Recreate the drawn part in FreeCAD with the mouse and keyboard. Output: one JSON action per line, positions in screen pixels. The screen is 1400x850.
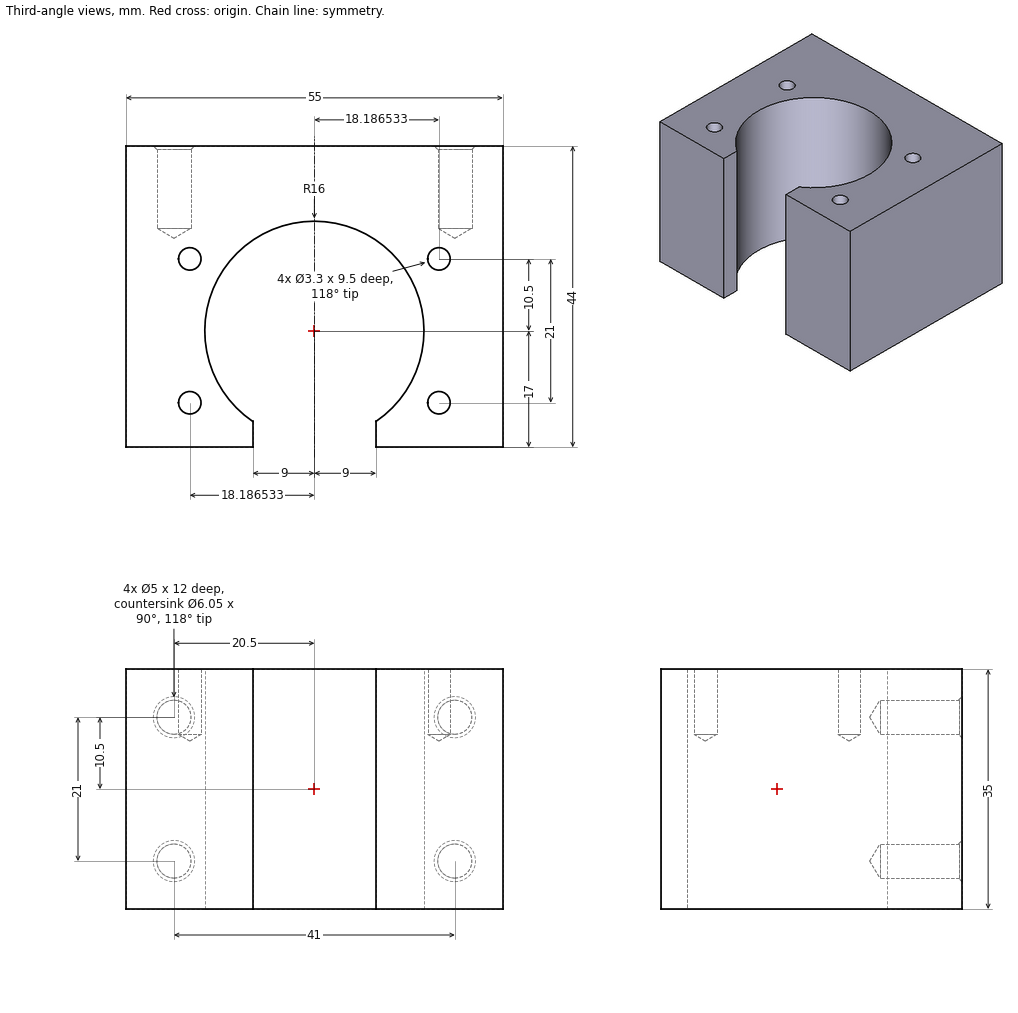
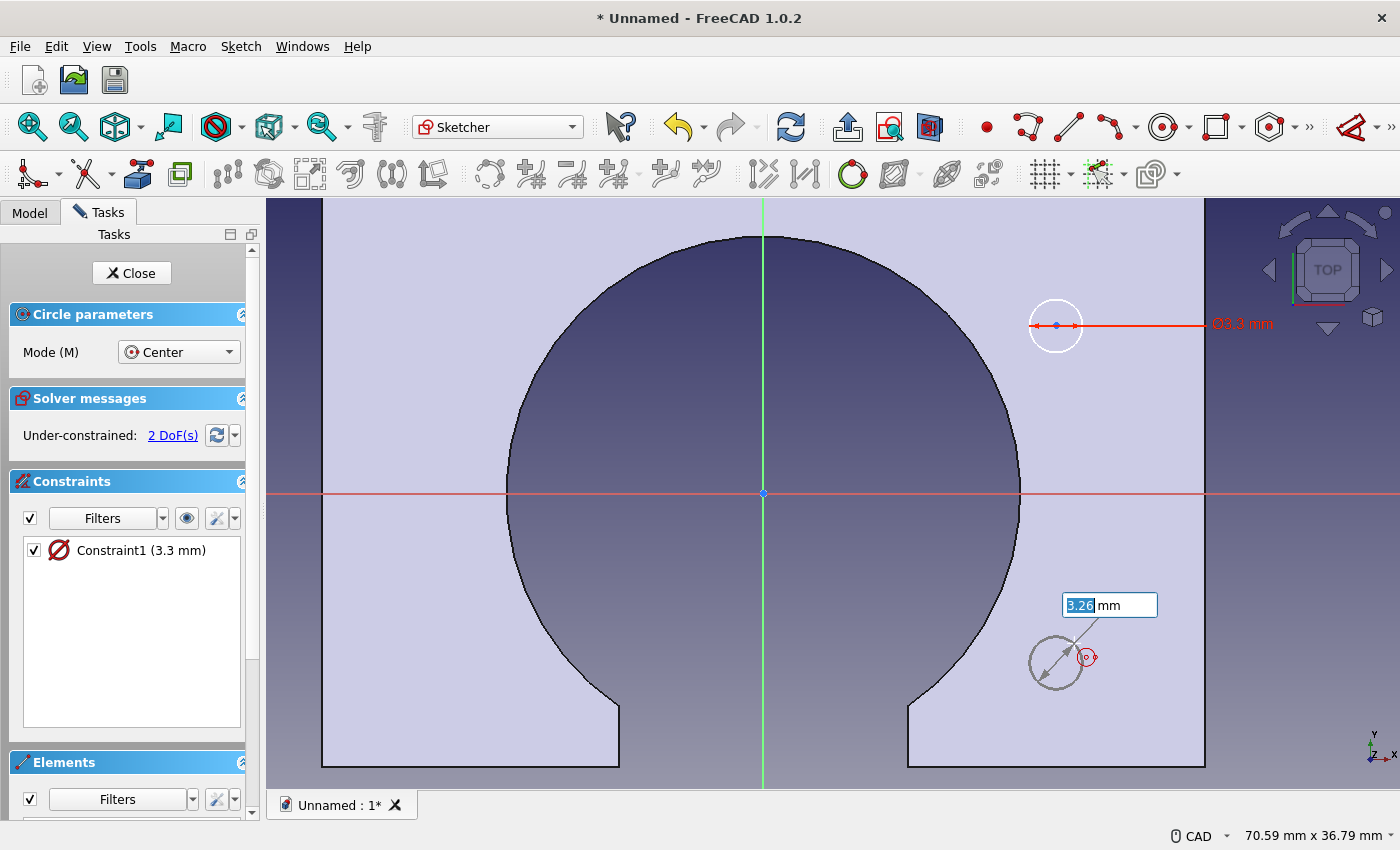
{"action": "type", "text": "3.3"}
{"action": "key", "text": "Return"}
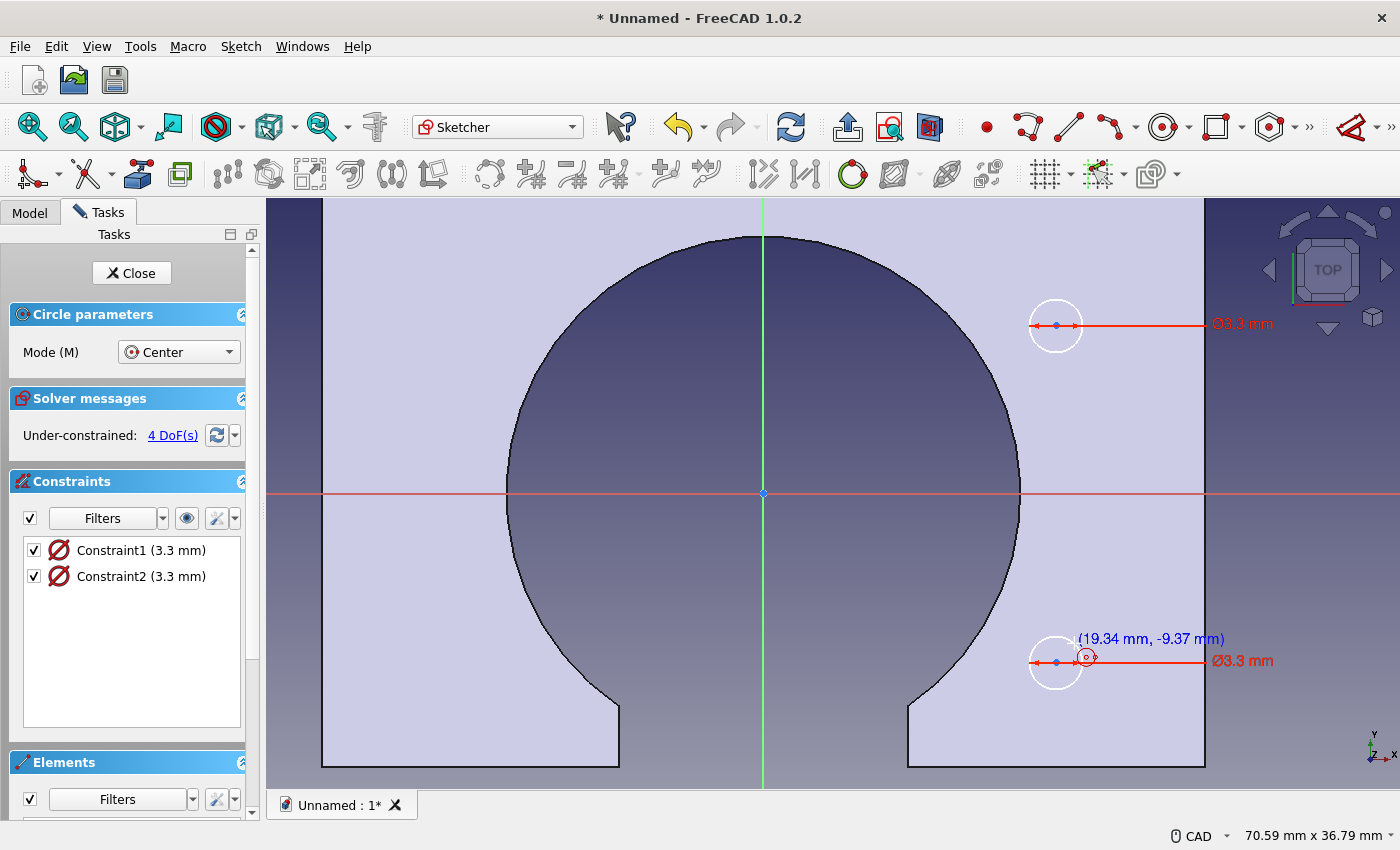
{"action": "left_click", "coordinate": [471, 662]}
{"action": "mouse_move", "coordinate": [490, 643]}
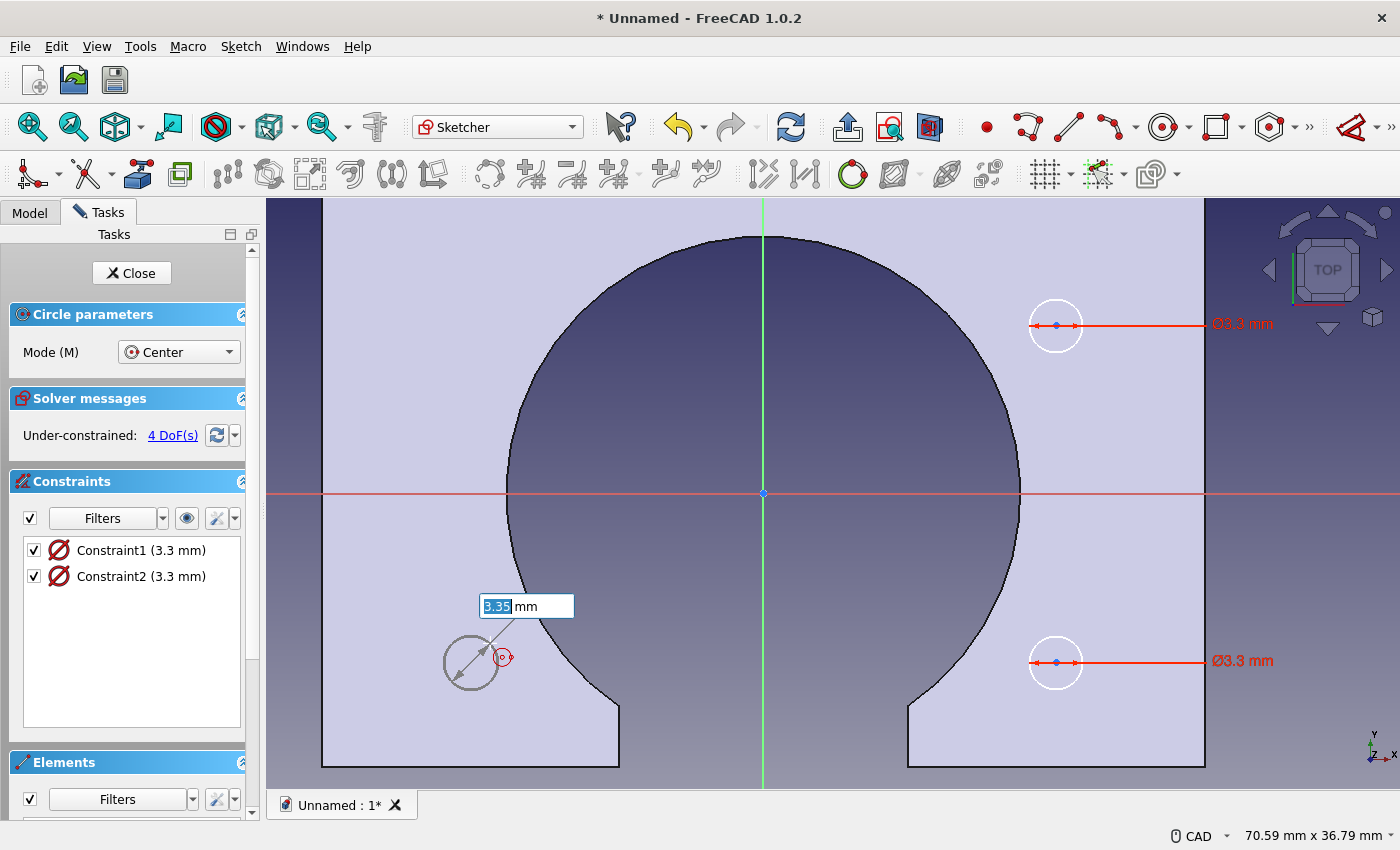
{"action": "type", "text": "3.3"}
{"action": "key", "text": "Return"}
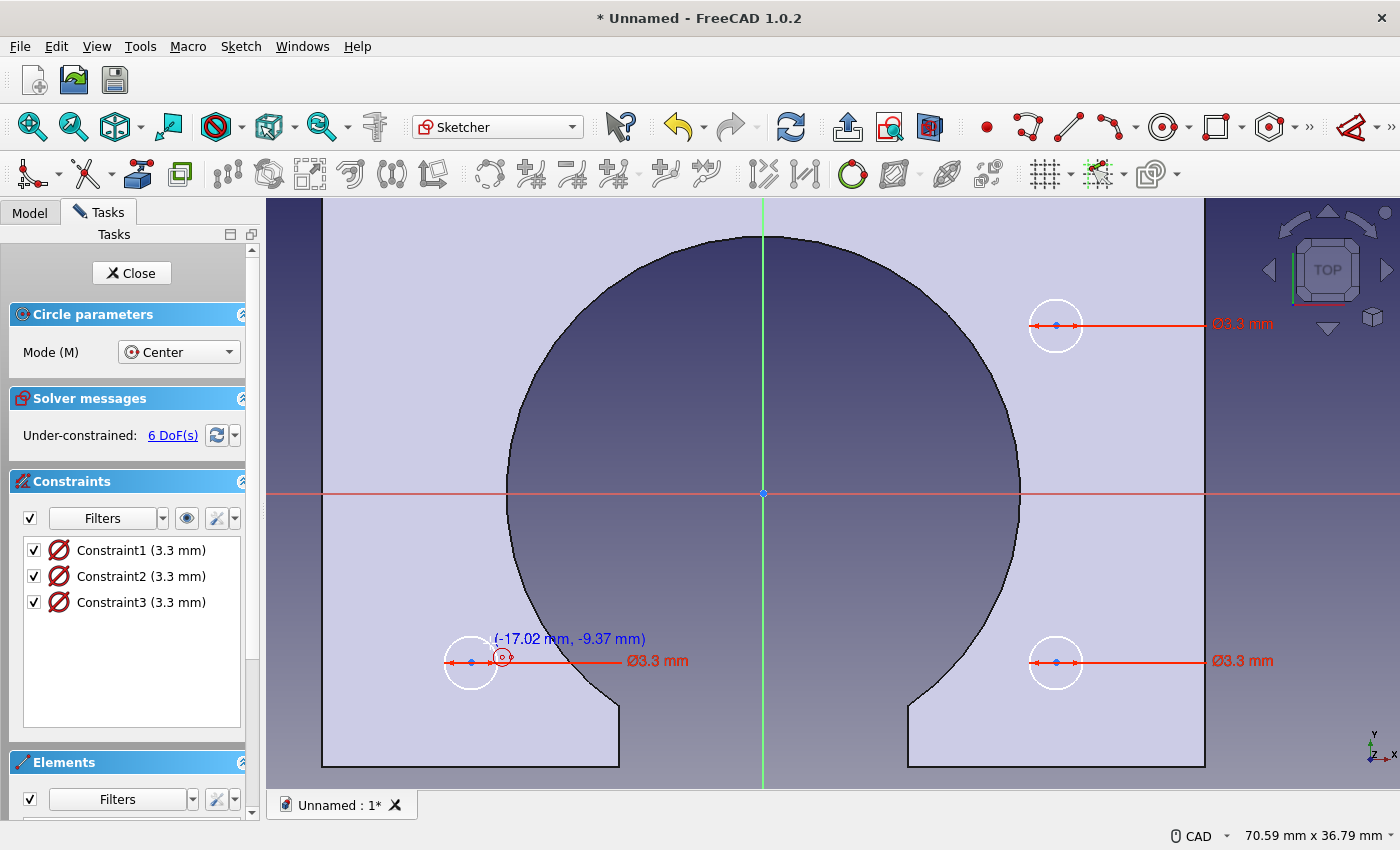
{"action": "left_click", "coordinate": [471, 325]}
{"action": "mouse_move", "coordinate": [490, 306]}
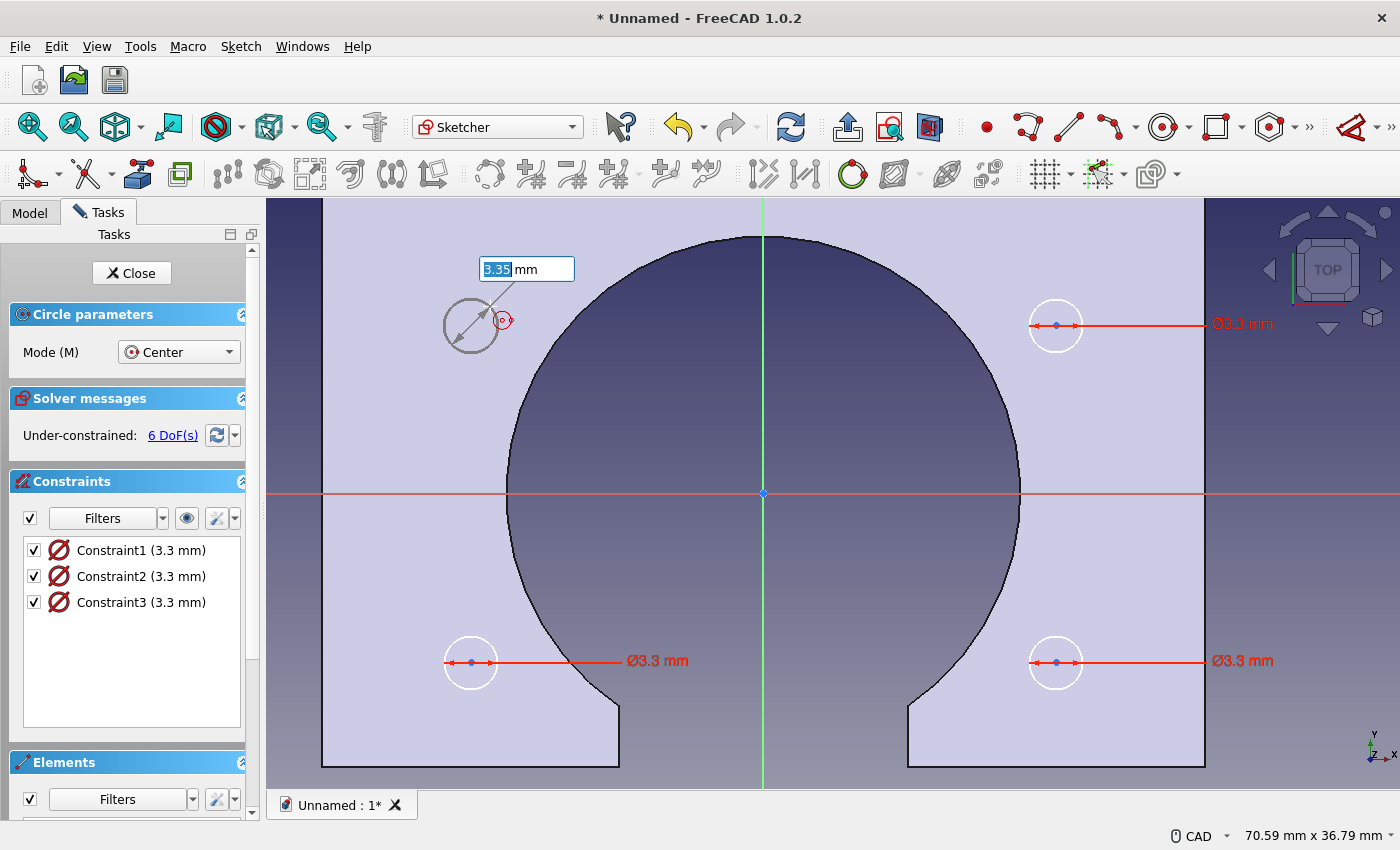
{"action": "type", "text": "3.3"}
{"action": "key", "text": "Return"}
{"action": "key", "text": "Escape"}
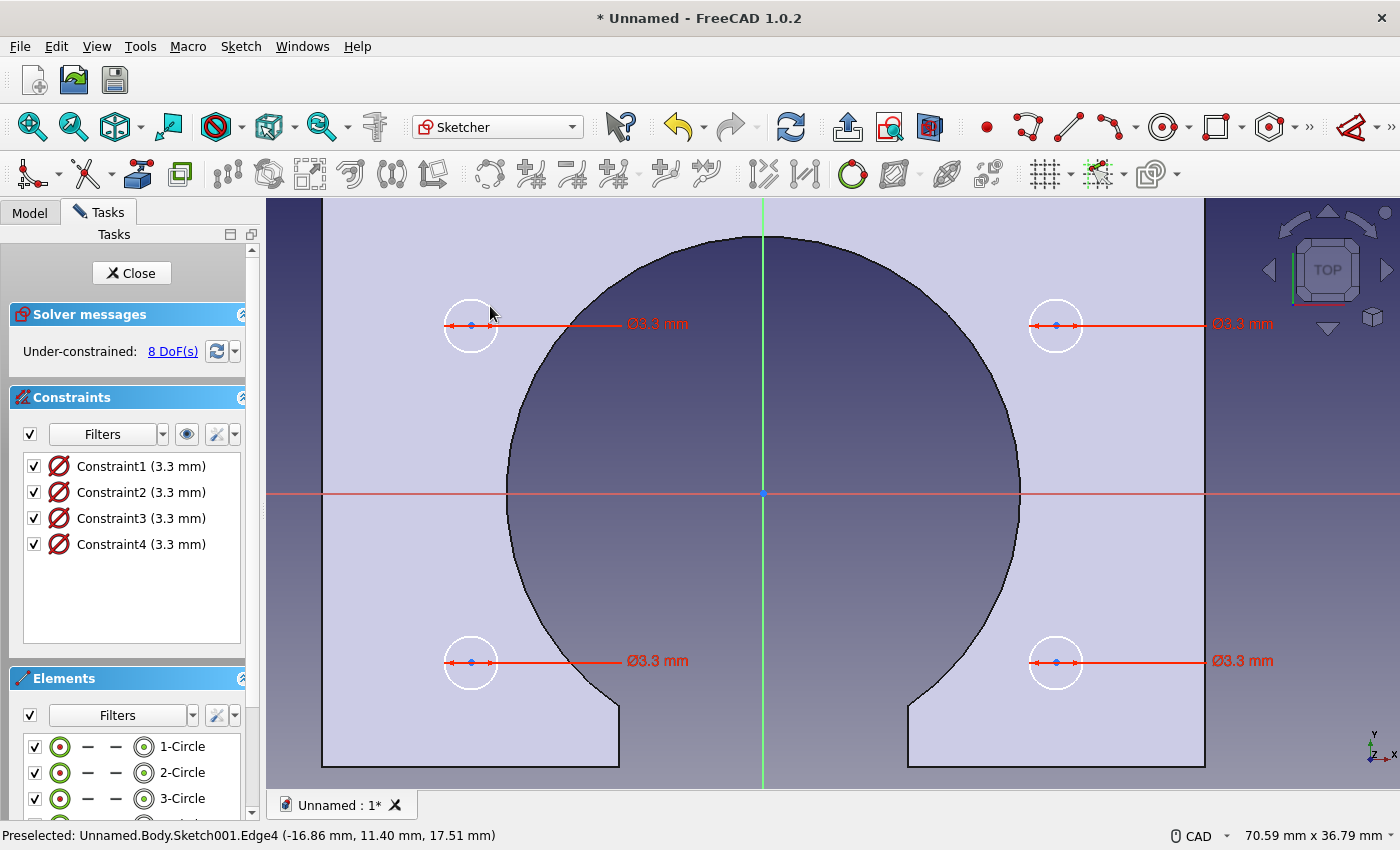
{"action": "left_click", "coordinate": [1056, 326]}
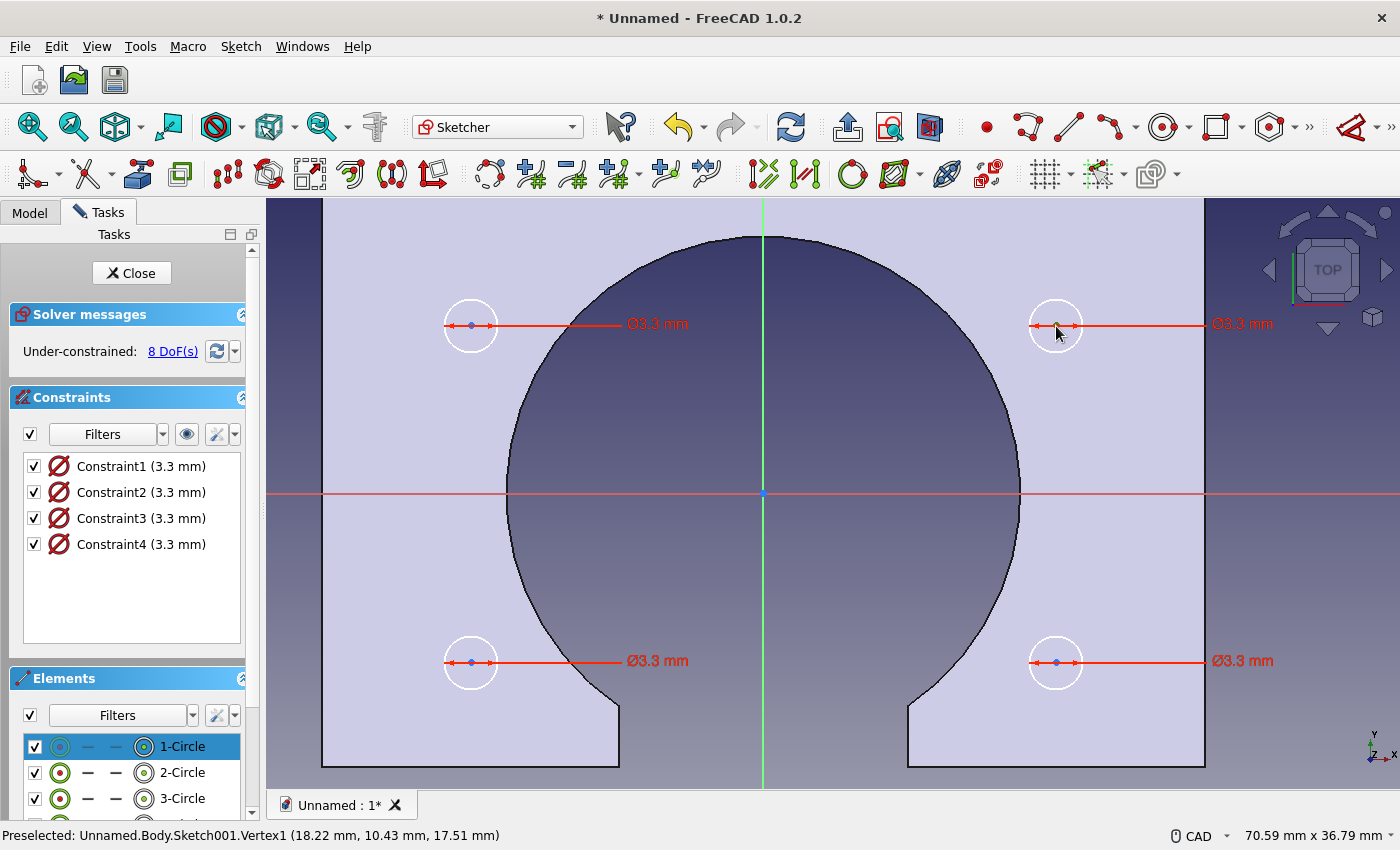
{"action": "left_click", "coordinate": [1056, 663]}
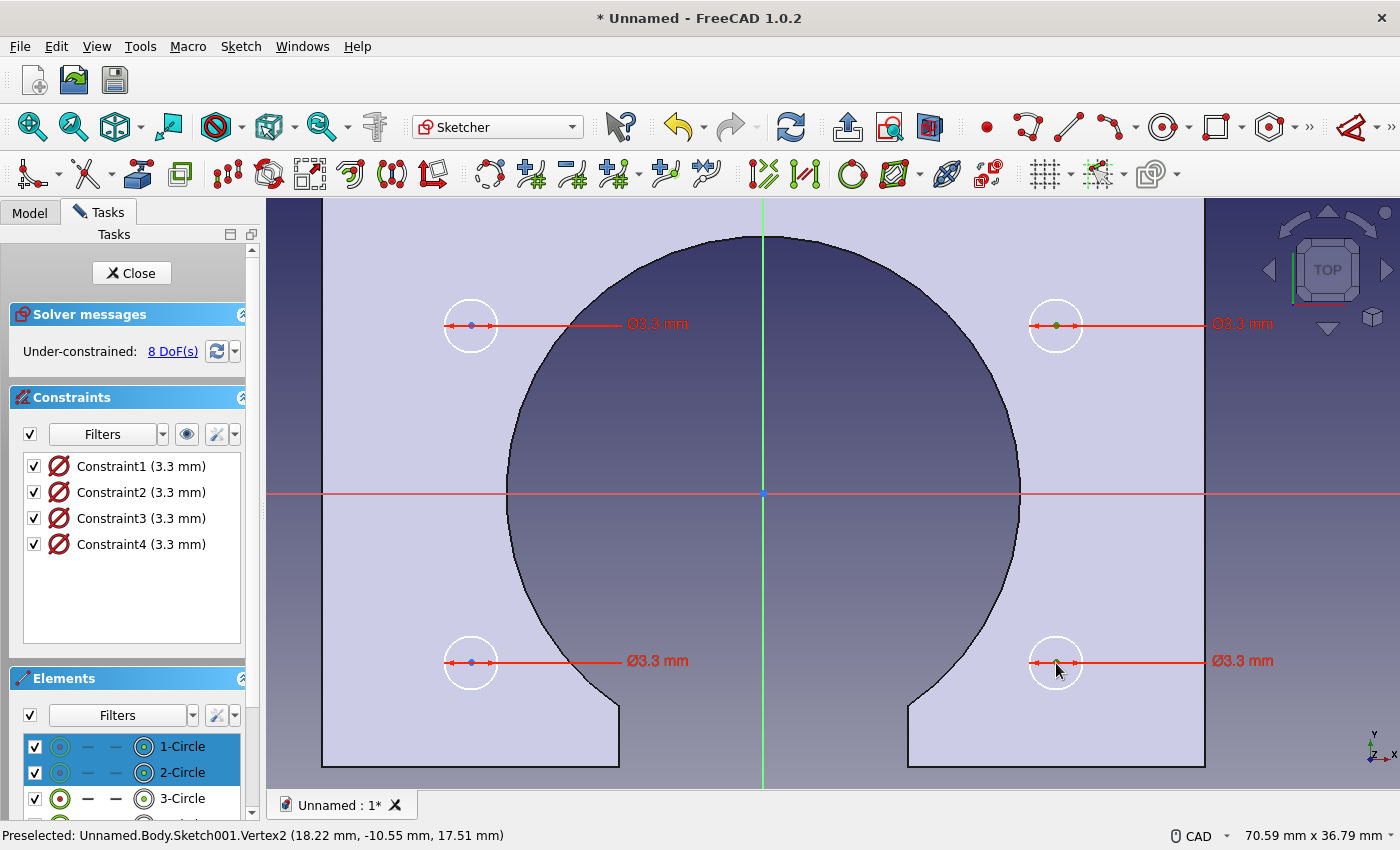
{"action": "key", "text": "v"}